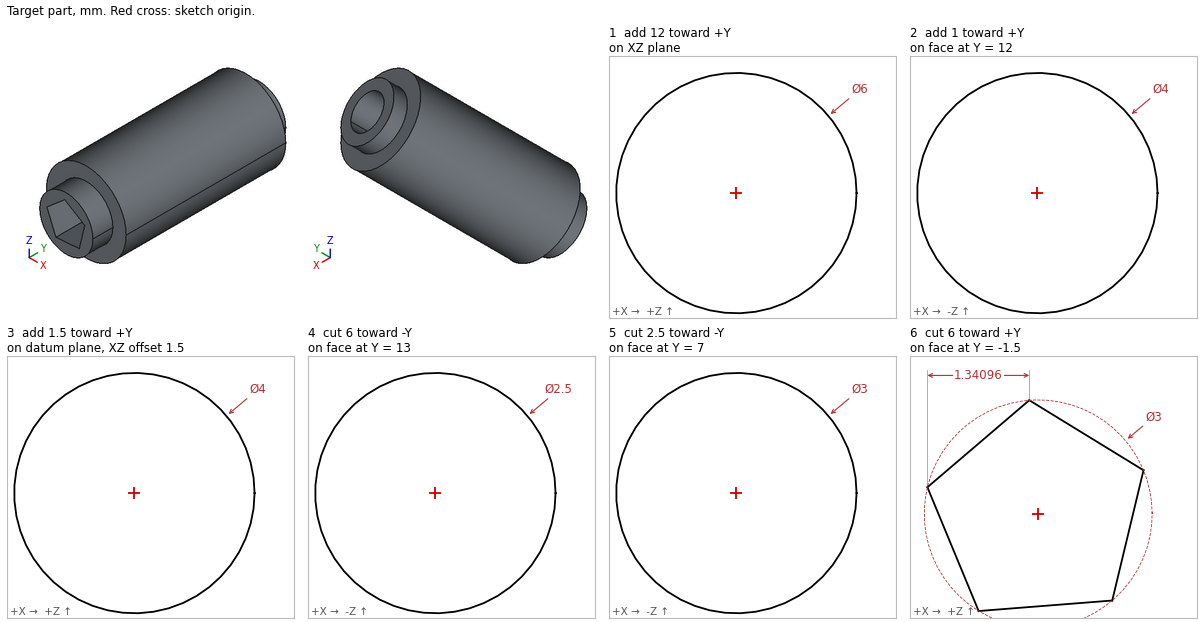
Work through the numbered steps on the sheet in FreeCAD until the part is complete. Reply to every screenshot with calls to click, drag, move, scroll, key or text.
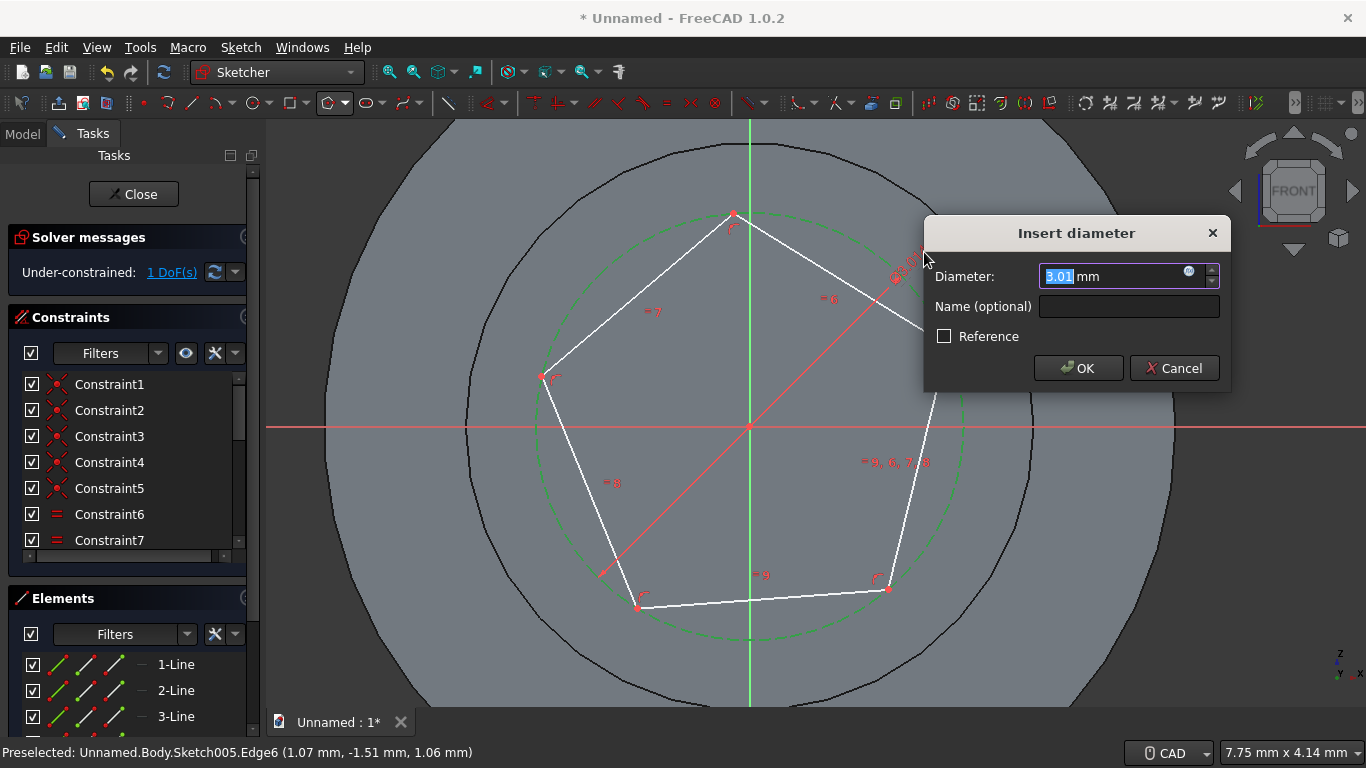
text(3)
key(Return)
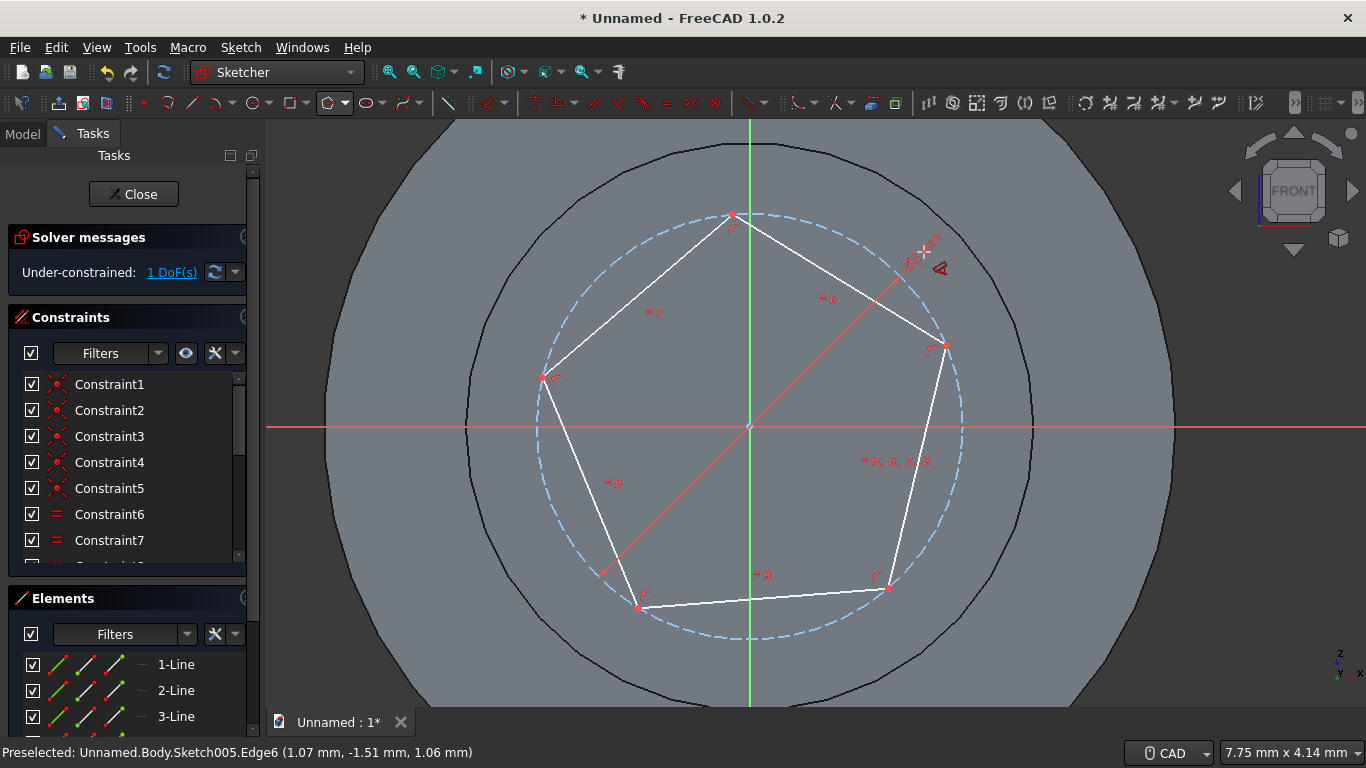
click(676, 263)
click(638, 180)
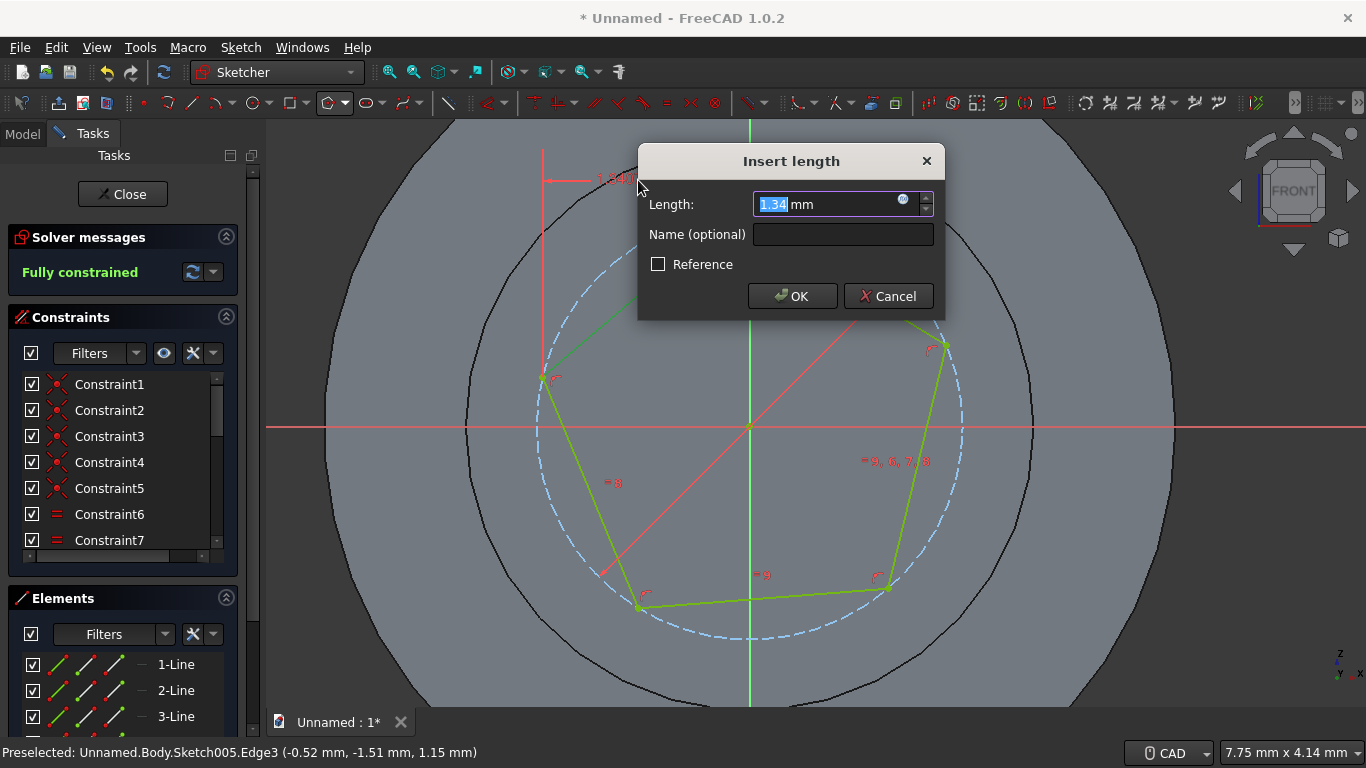
text(1.34096)
key(Return)
key(Escape)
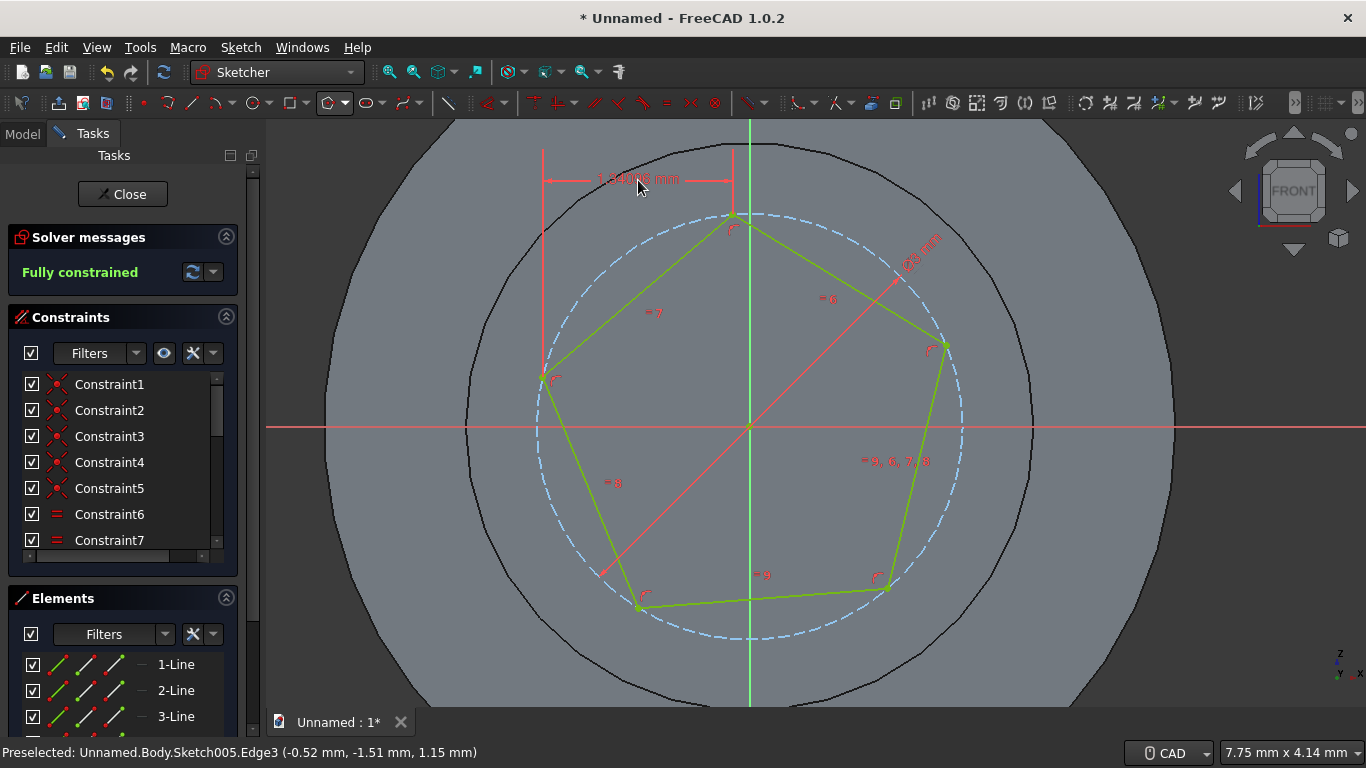
click(123, 194)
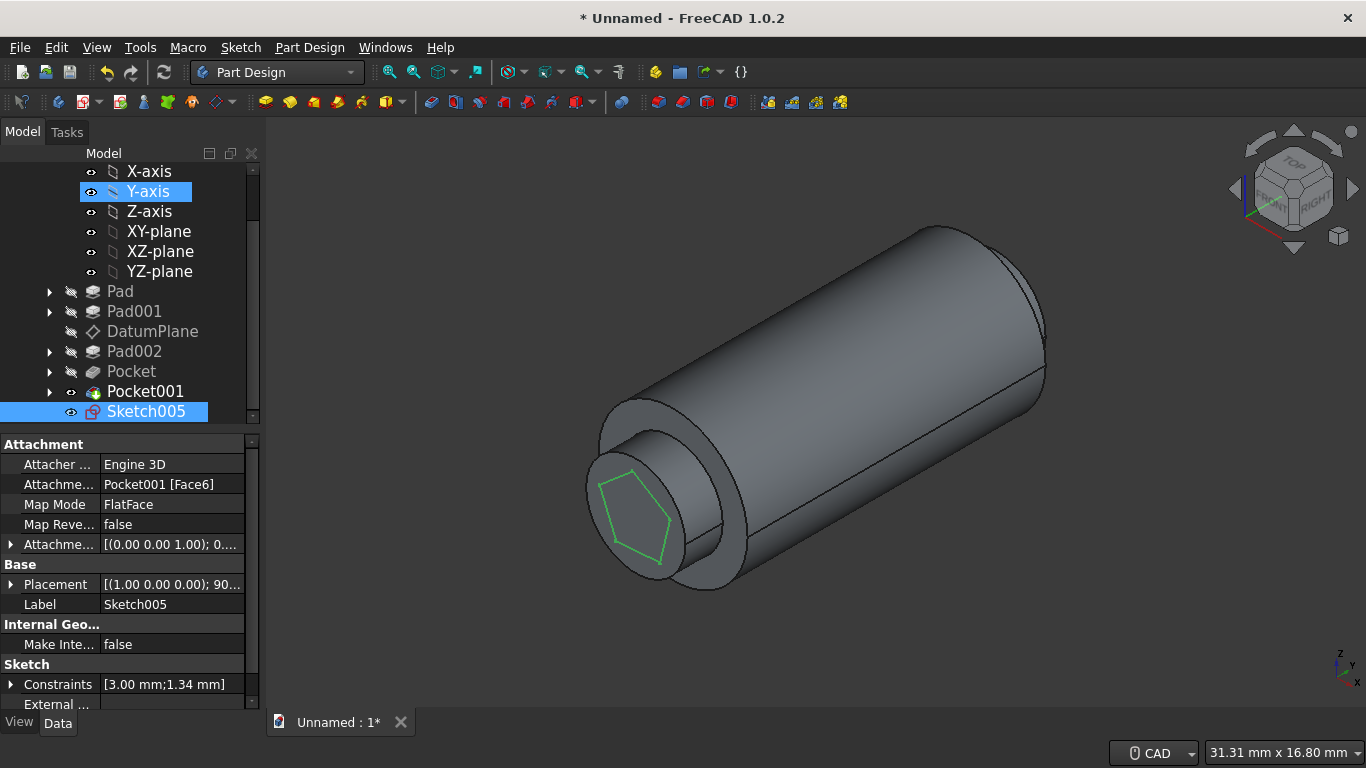
click(432, 102)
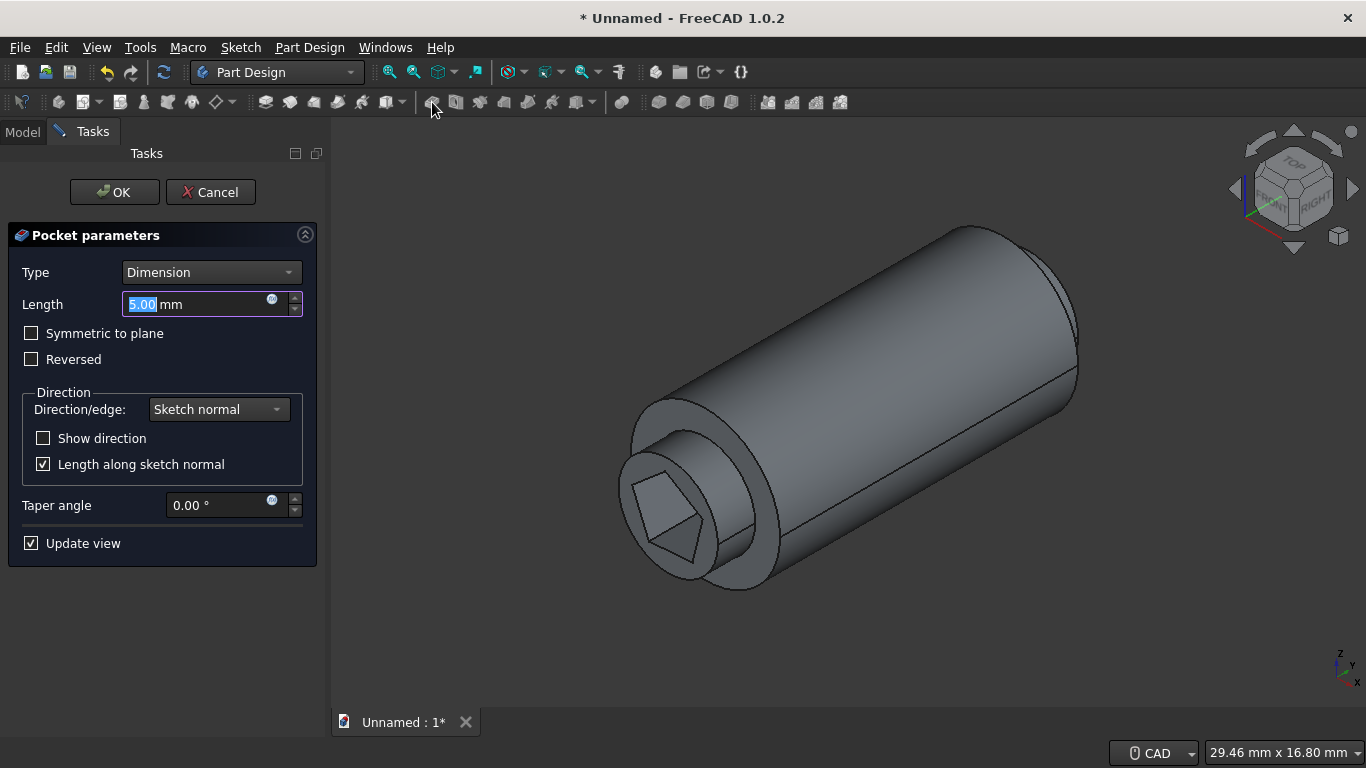
text(6)
key(Tab)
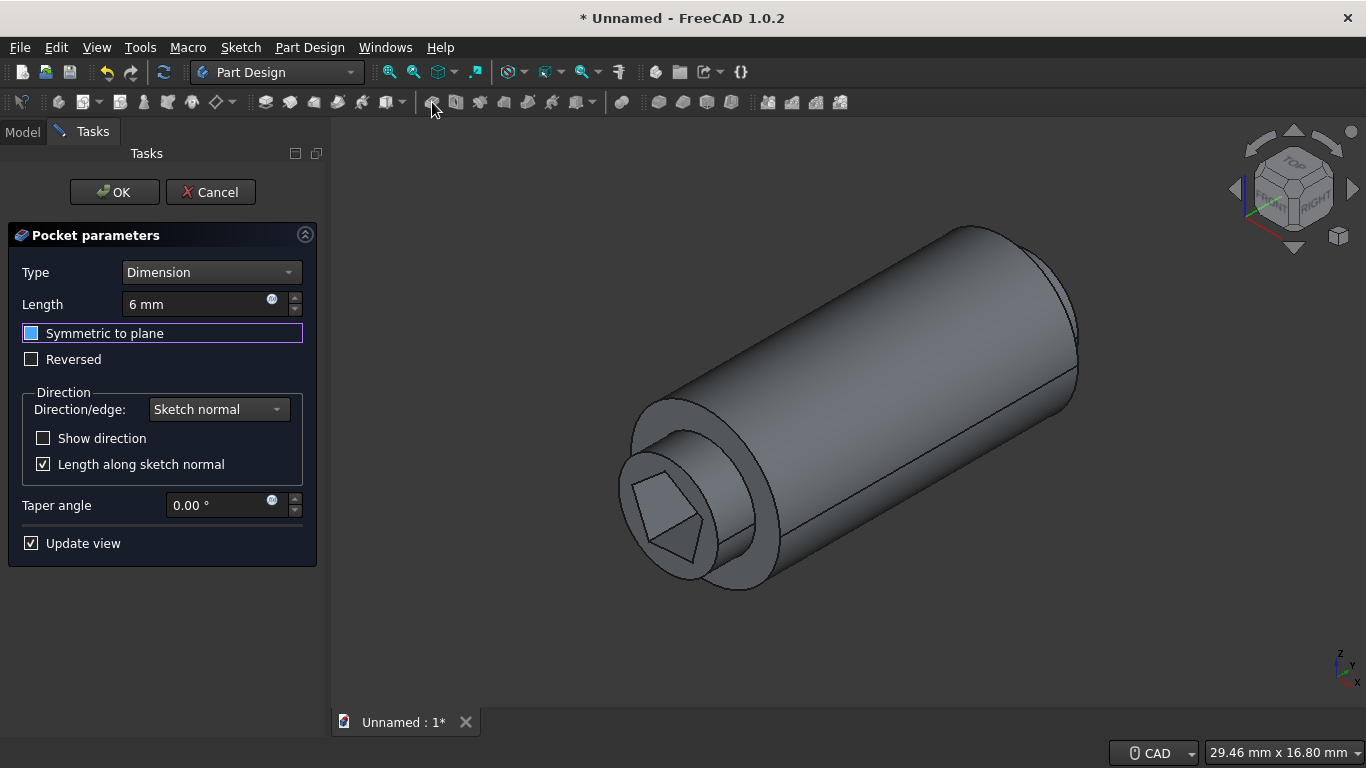
click(115, 192)